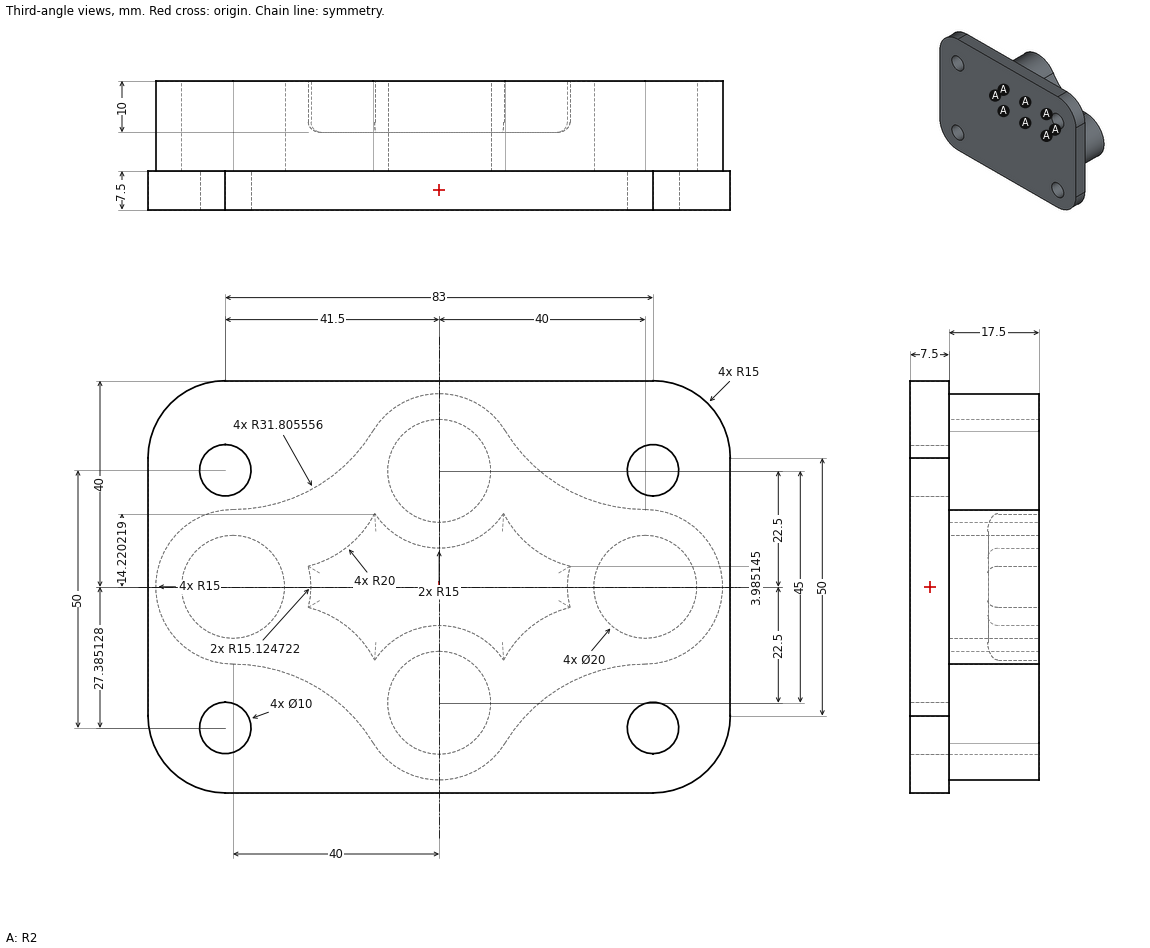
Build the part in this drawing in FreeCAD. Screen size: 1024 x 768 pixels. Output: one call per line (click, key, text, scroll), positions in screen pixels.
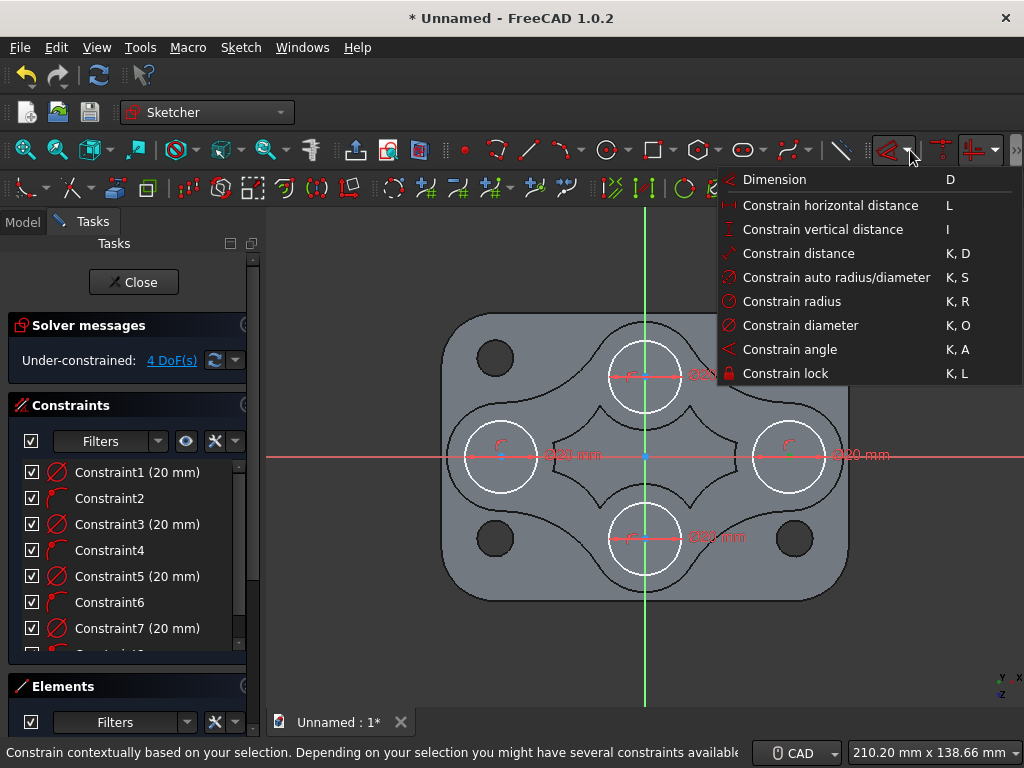
click(870, 205)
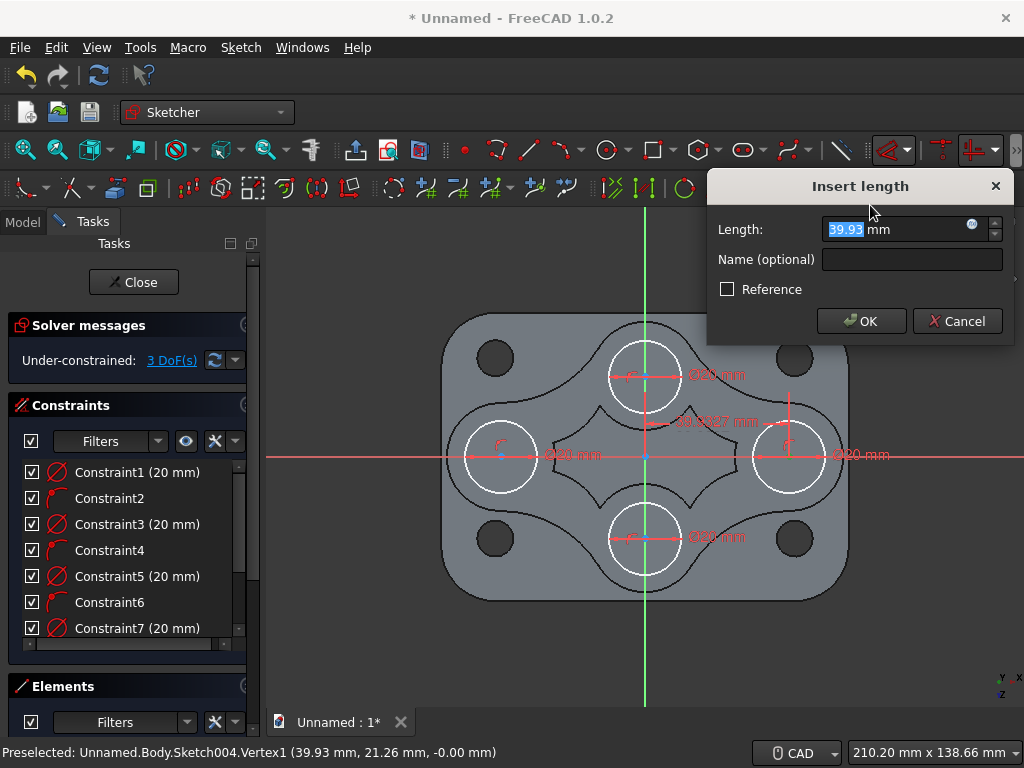
text(40)
key(Return)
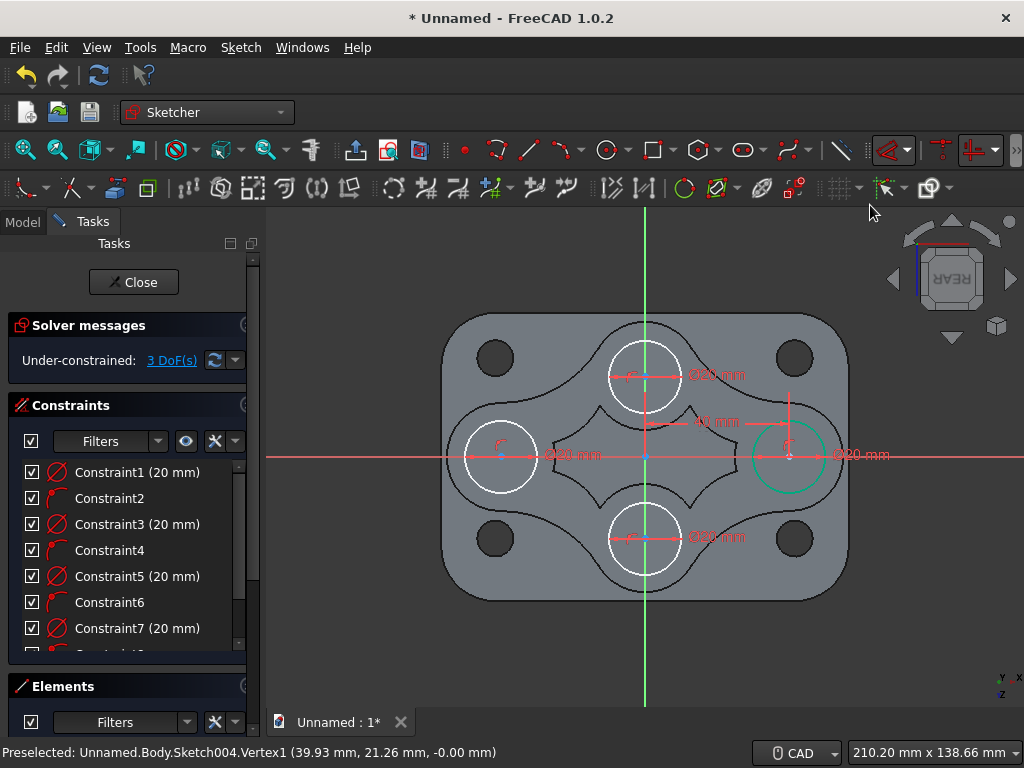
click(501, 457)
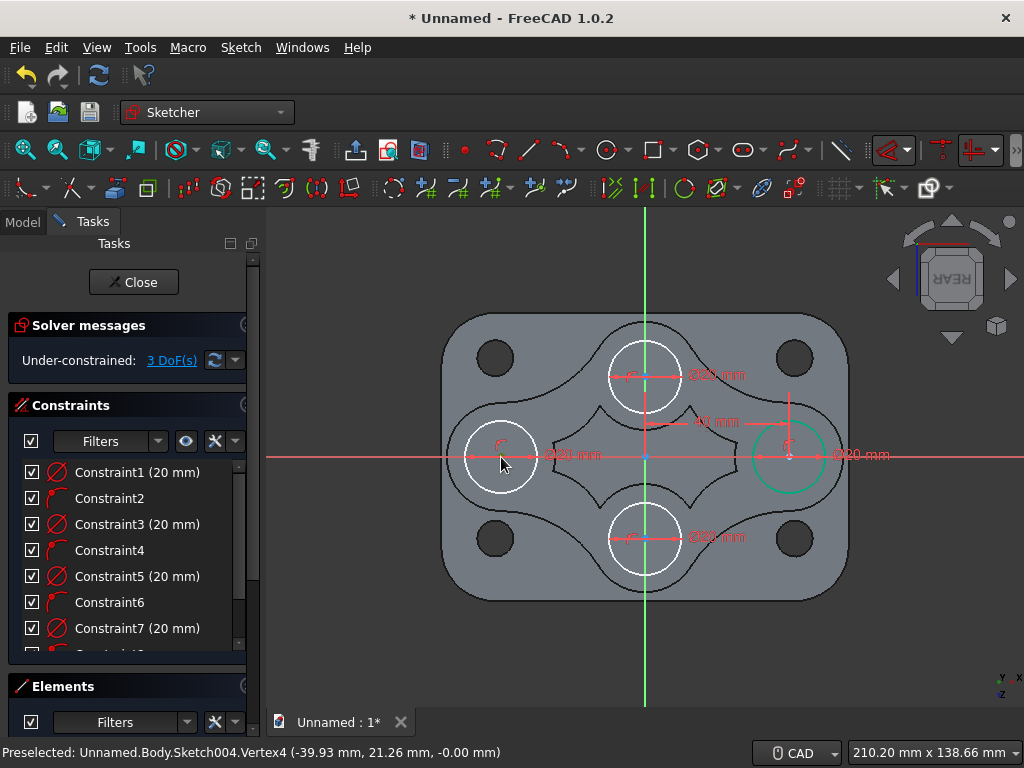
key(l)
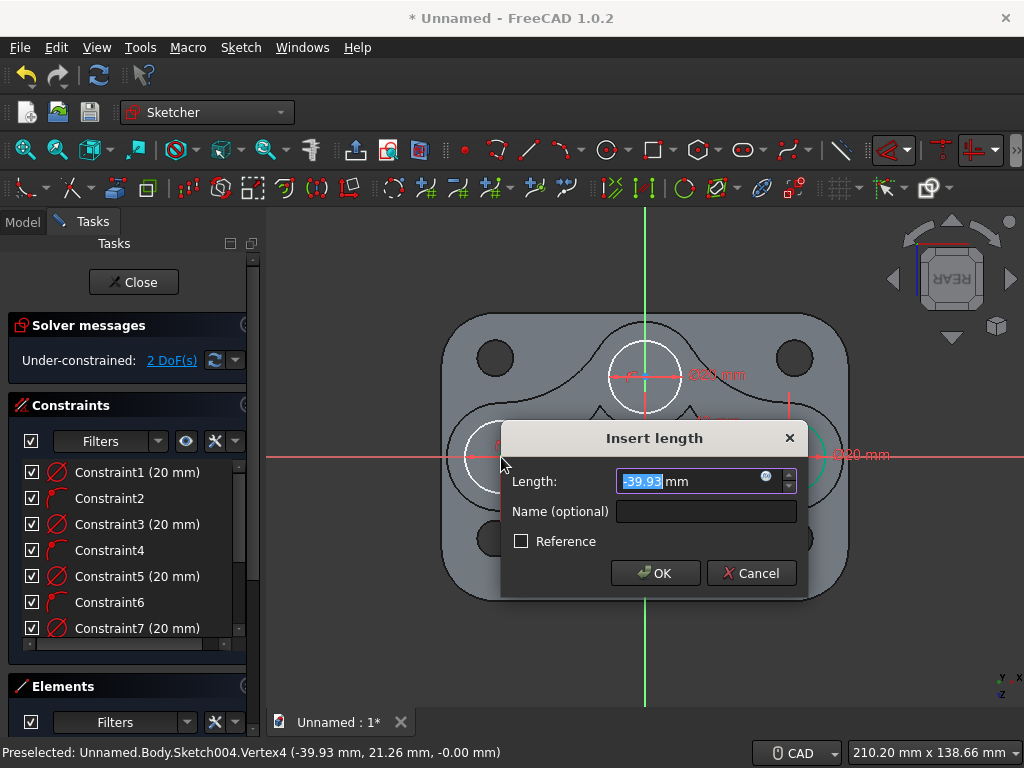
text(-40)
key(Return)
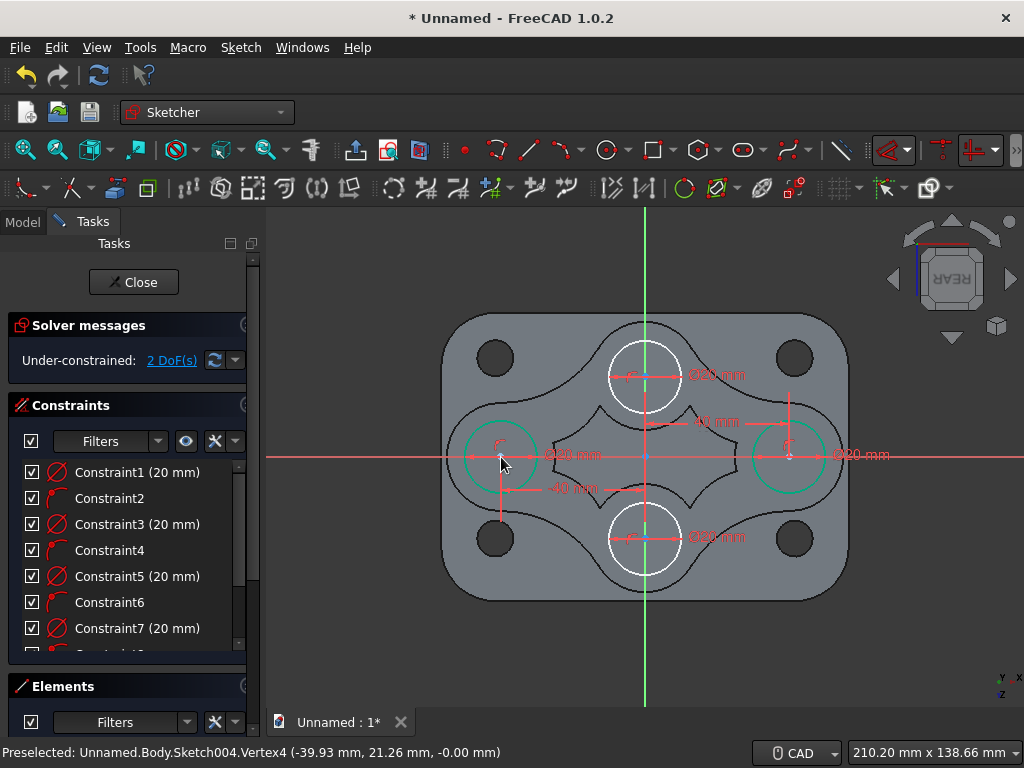
click(645, 539)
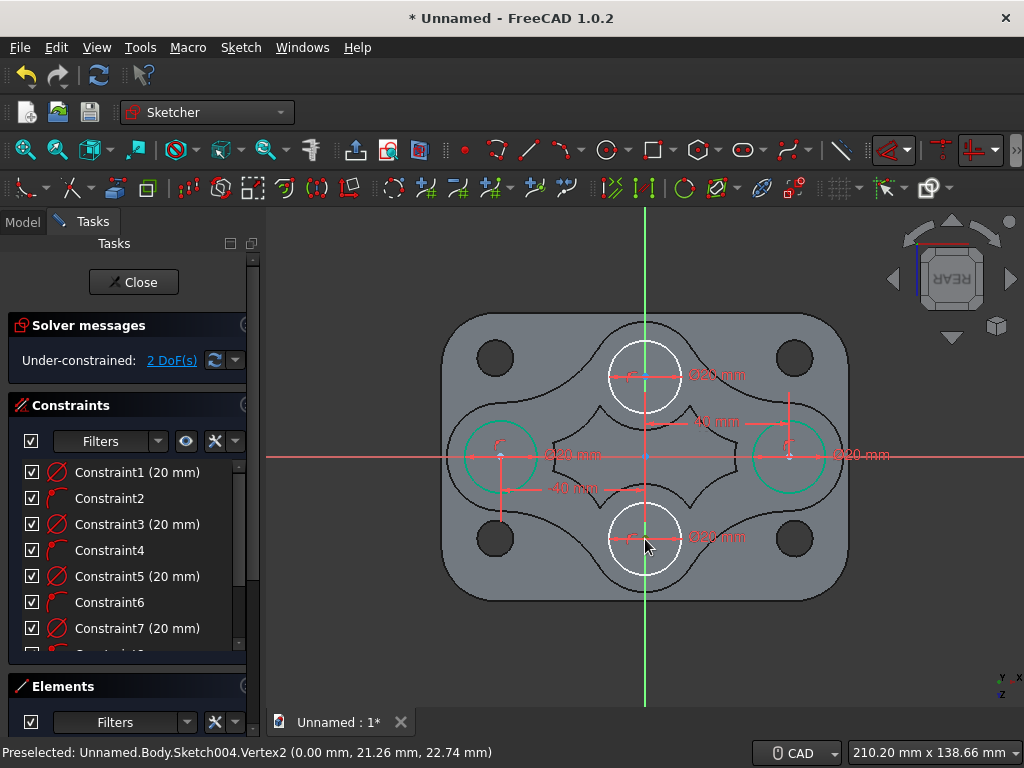
click(645, 377)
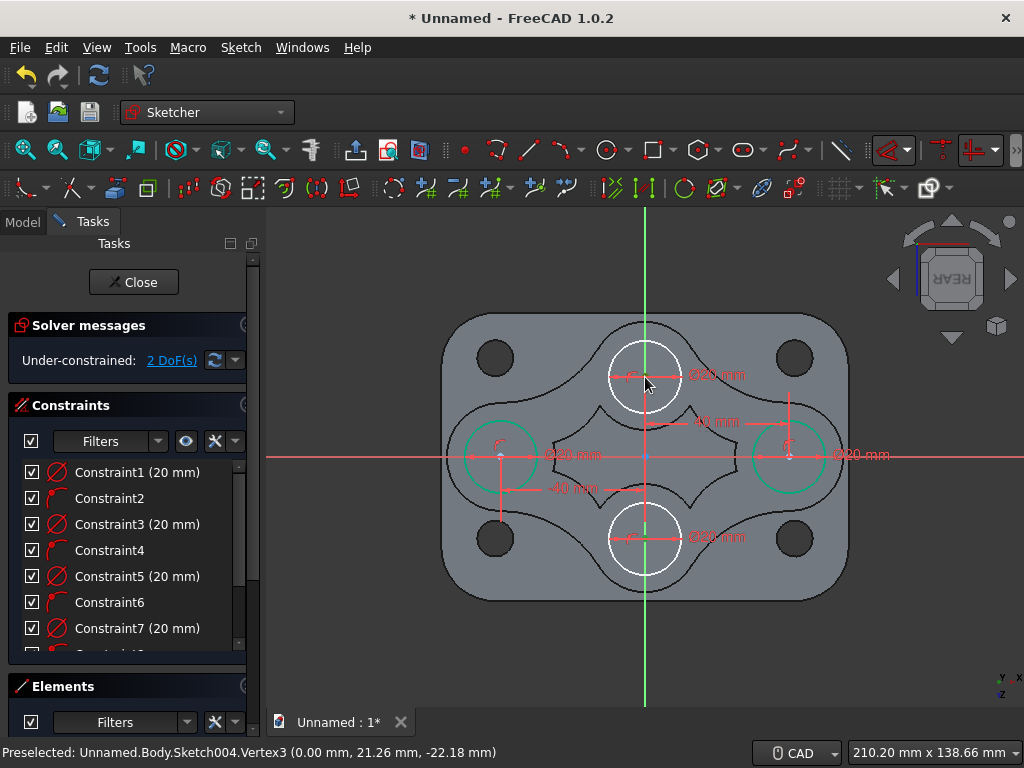
click(910, 150)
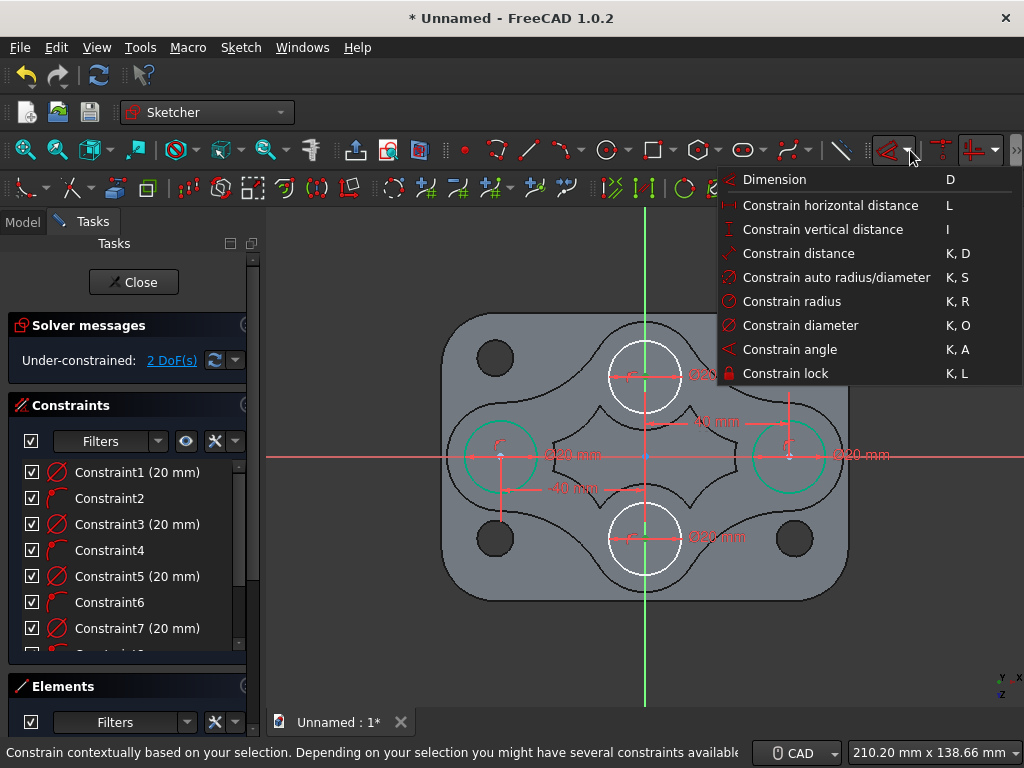
click(870, 229)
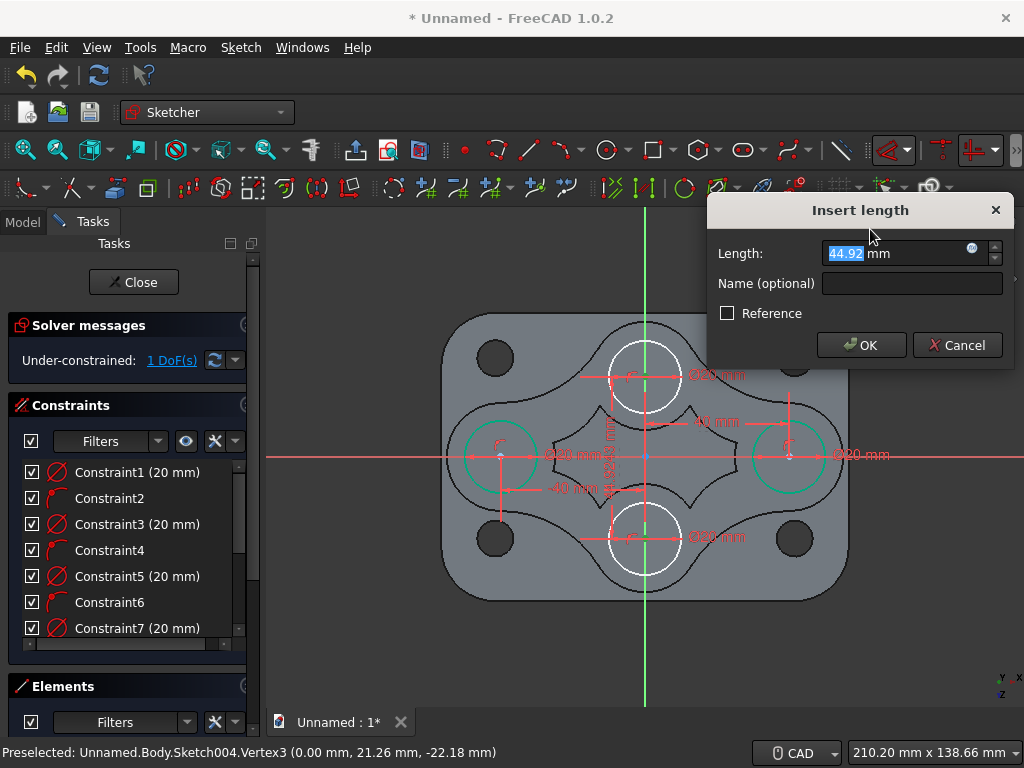
text(45)
key(Return)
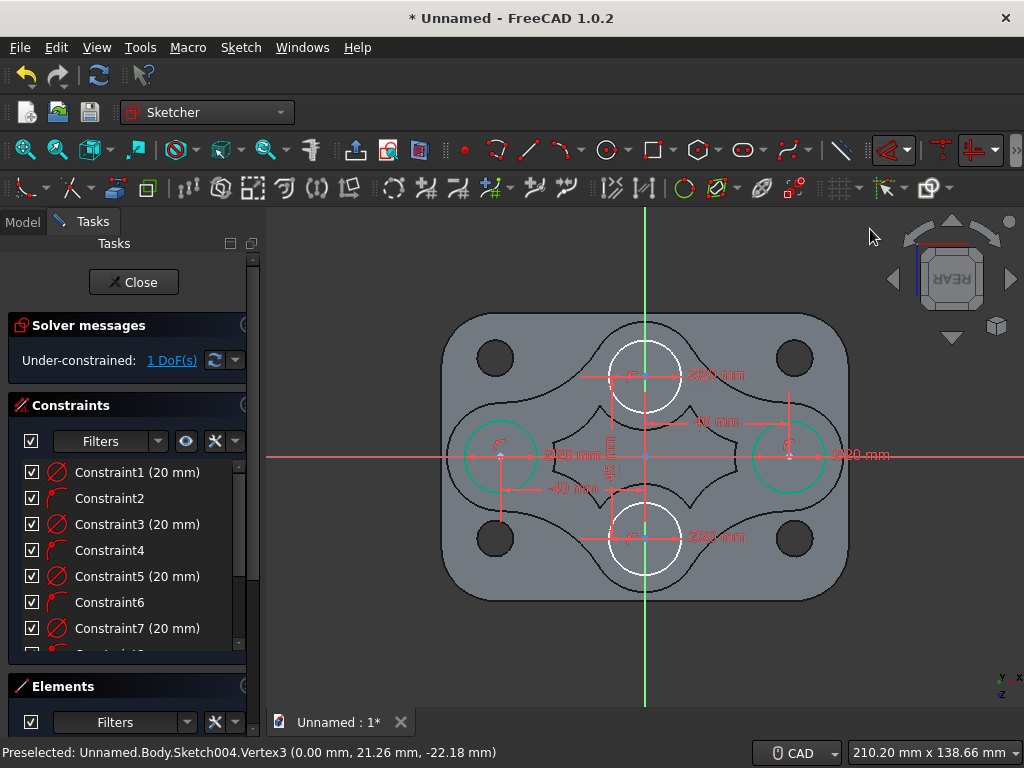
click(645, 539)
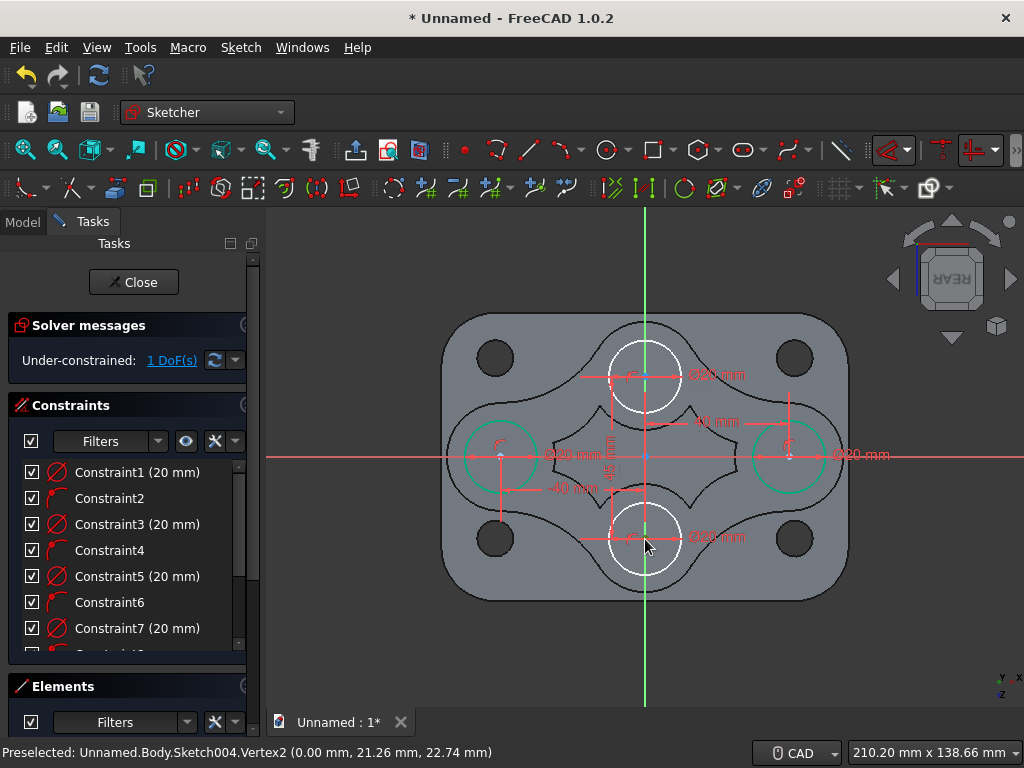
click(910, 150)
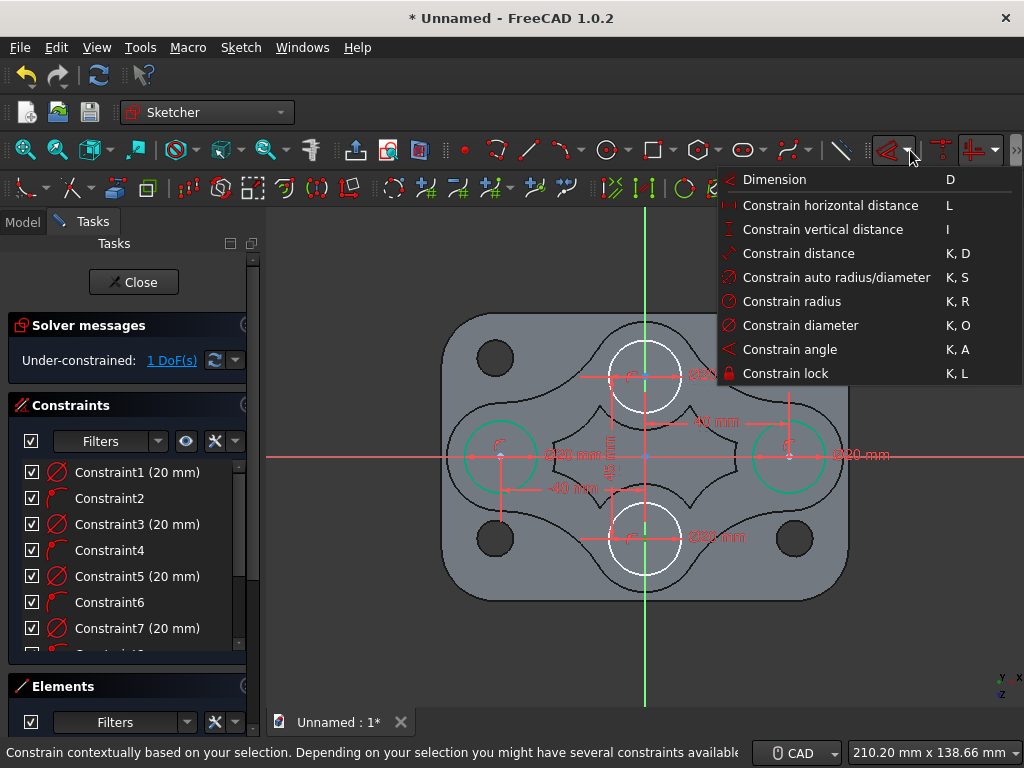
click(870, 229)